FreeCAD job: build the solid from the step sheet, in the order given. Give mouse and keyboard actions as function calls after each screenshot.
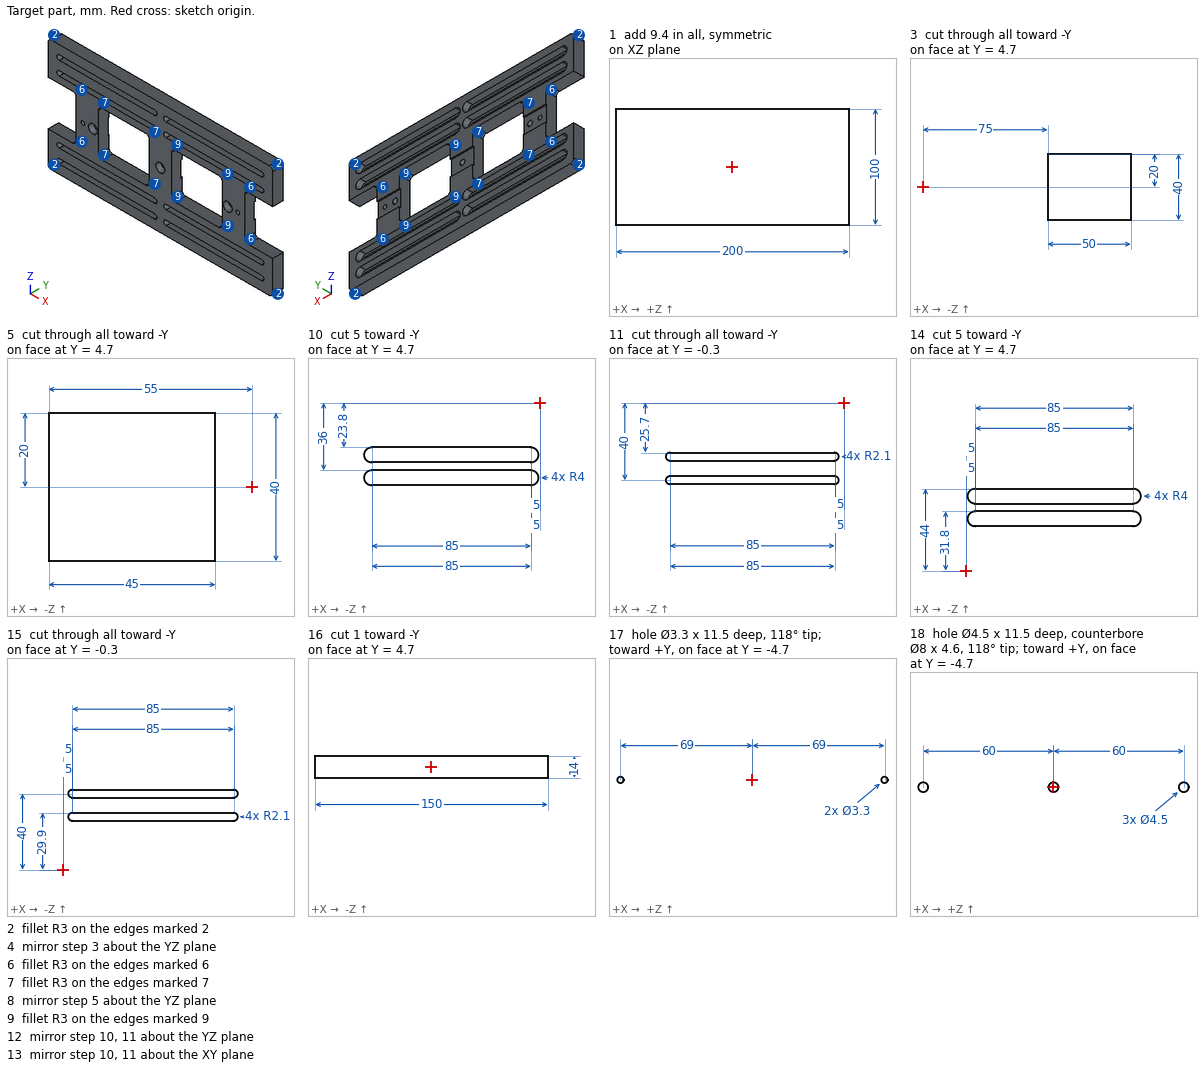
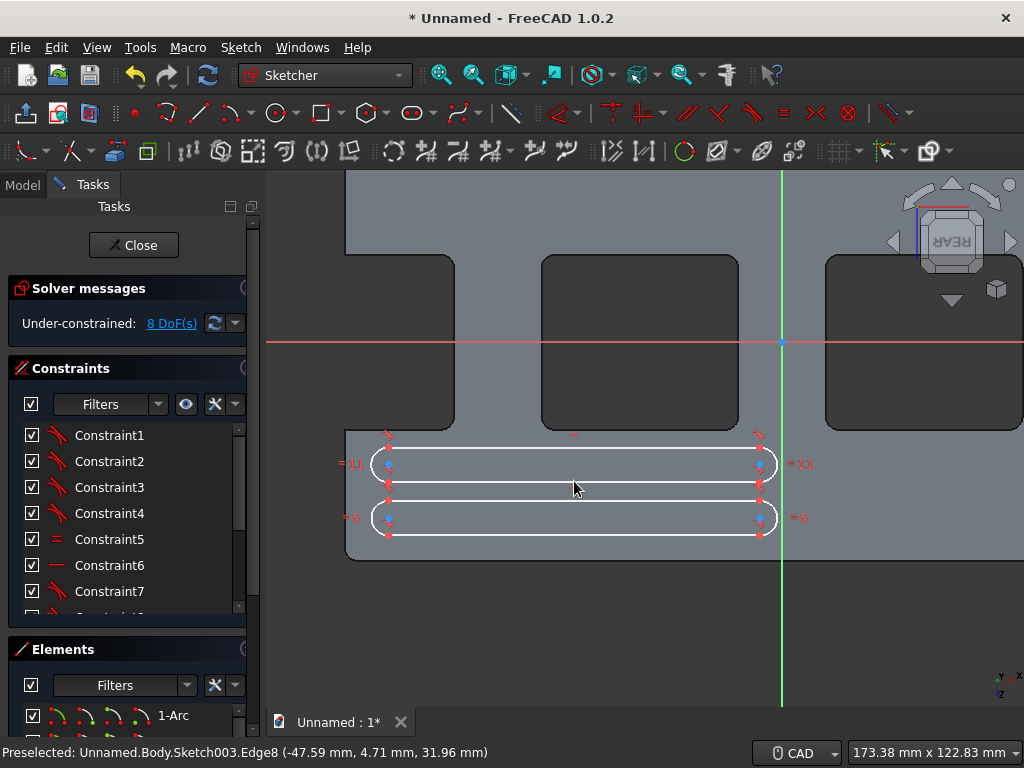
click(375, 508)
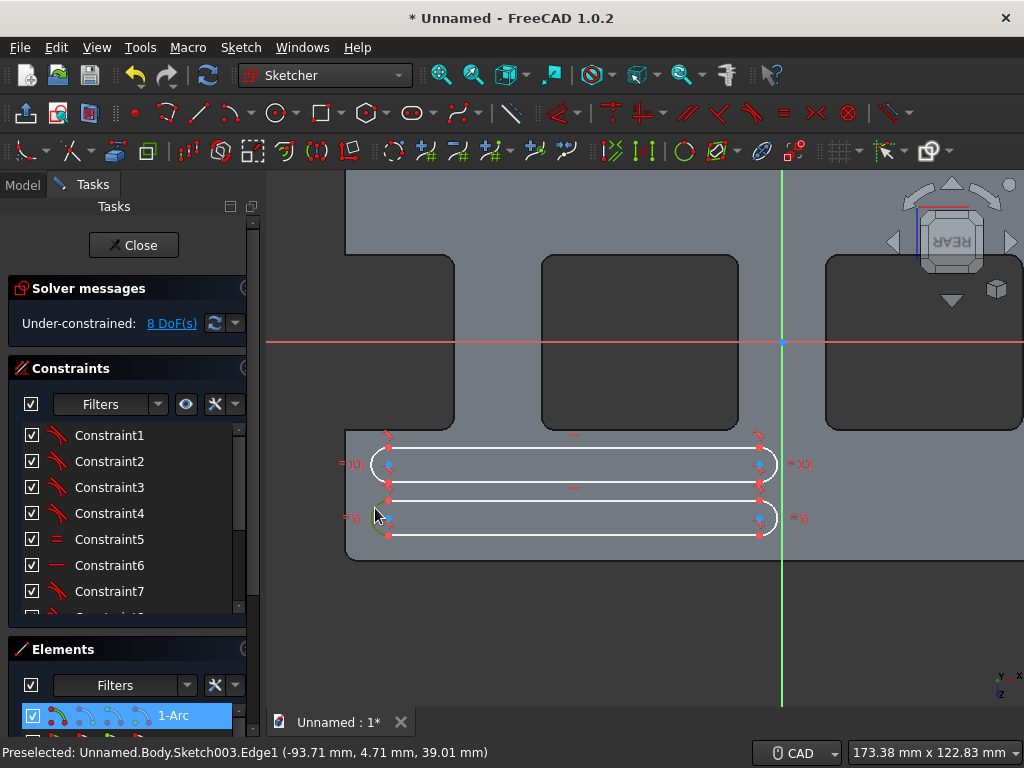
click(375, 455)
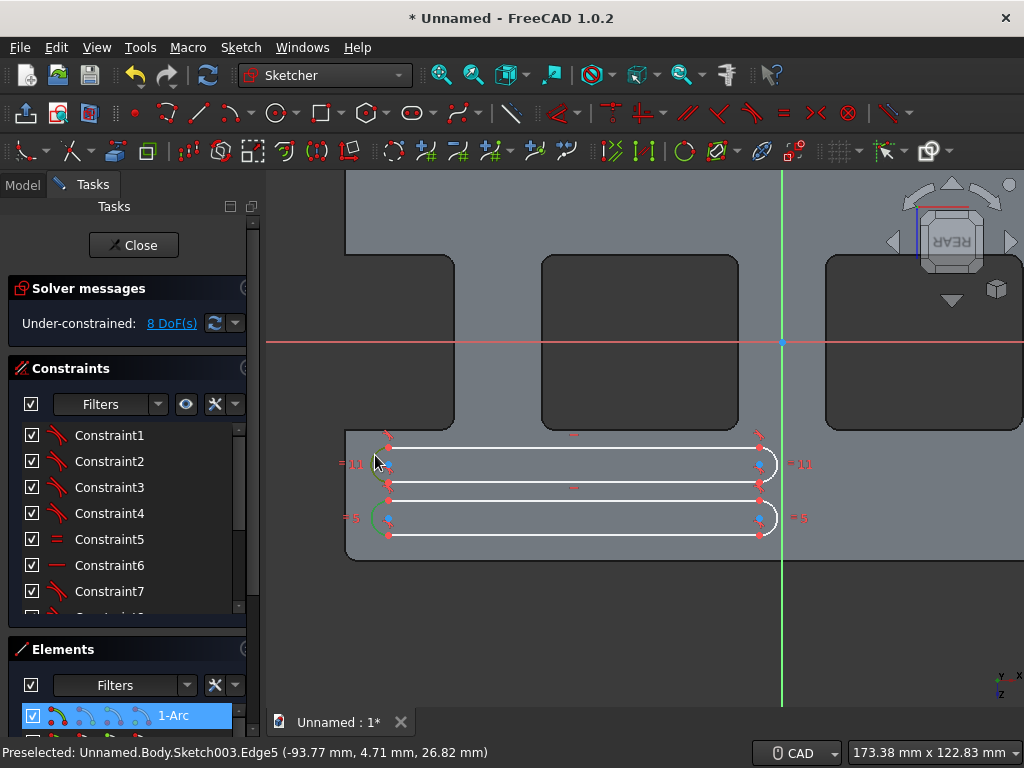
click(784, 114)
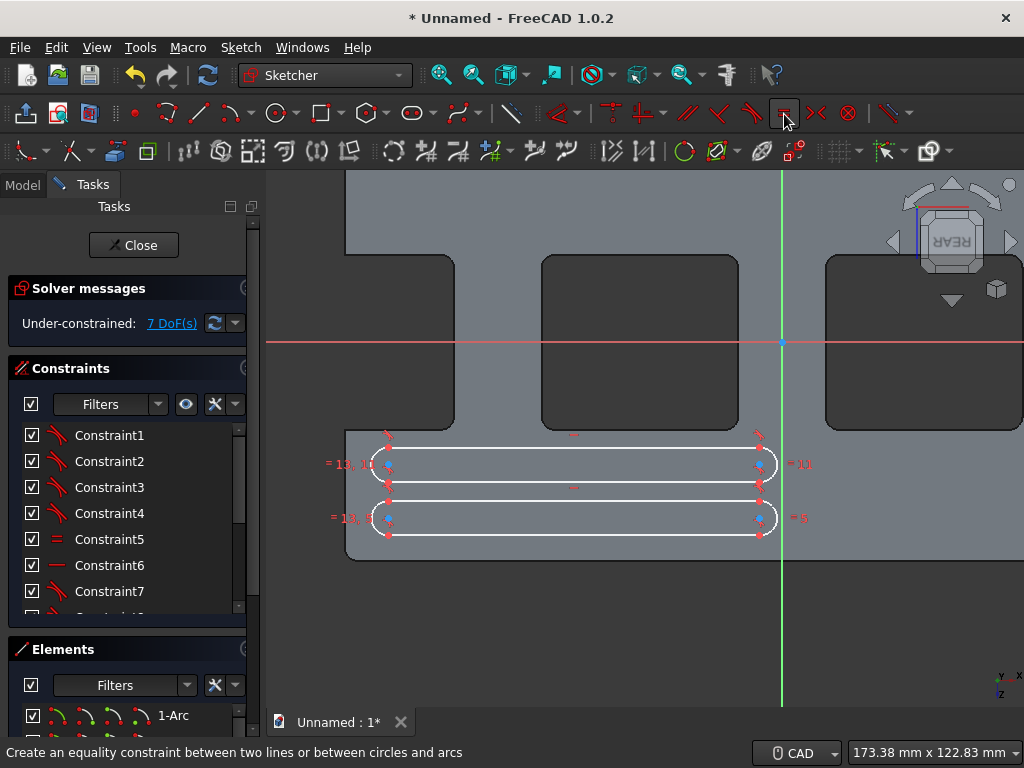
key(d)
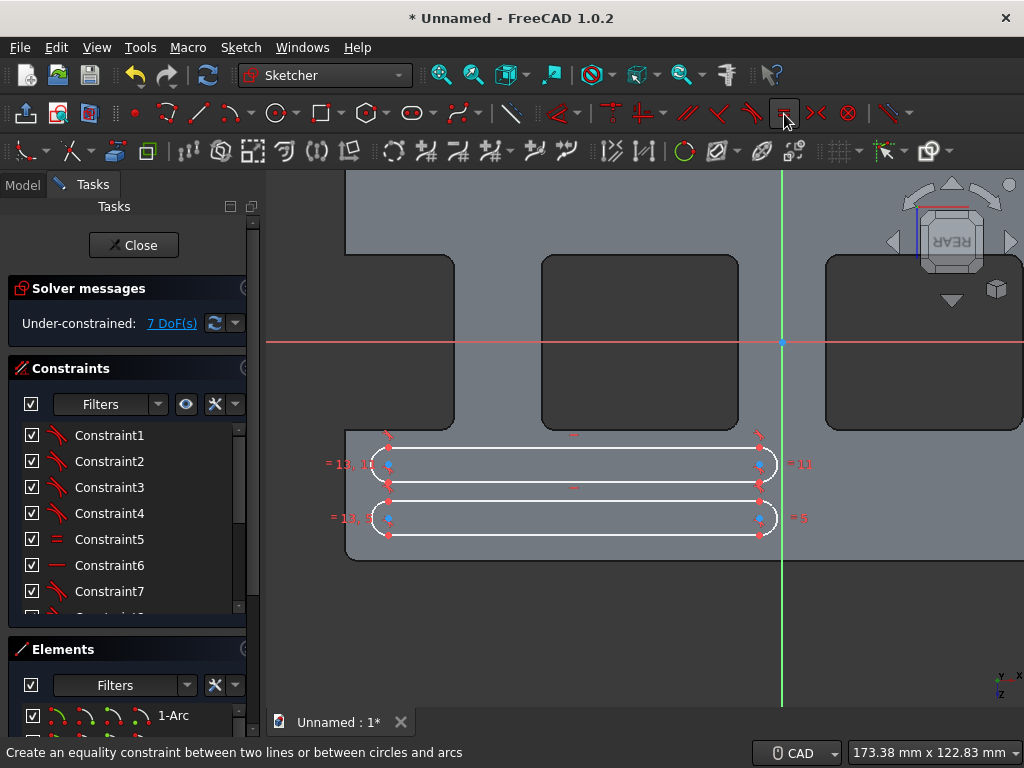
scroll(375, 508, up, 5)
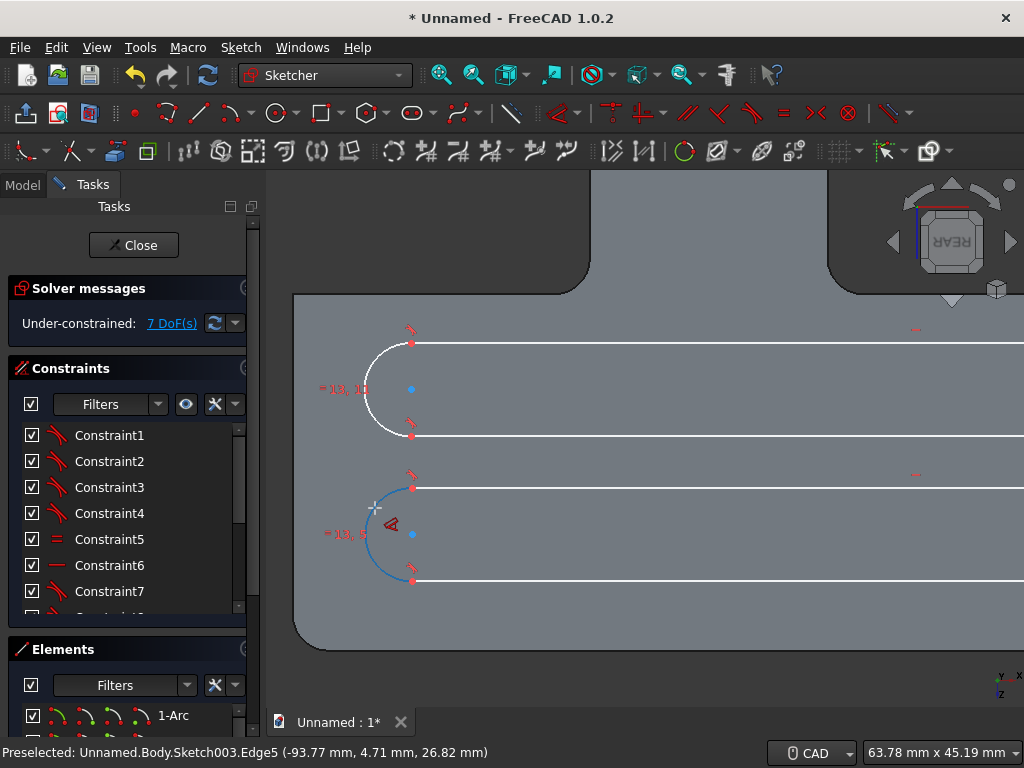
click(374, 507)
click(348, 488)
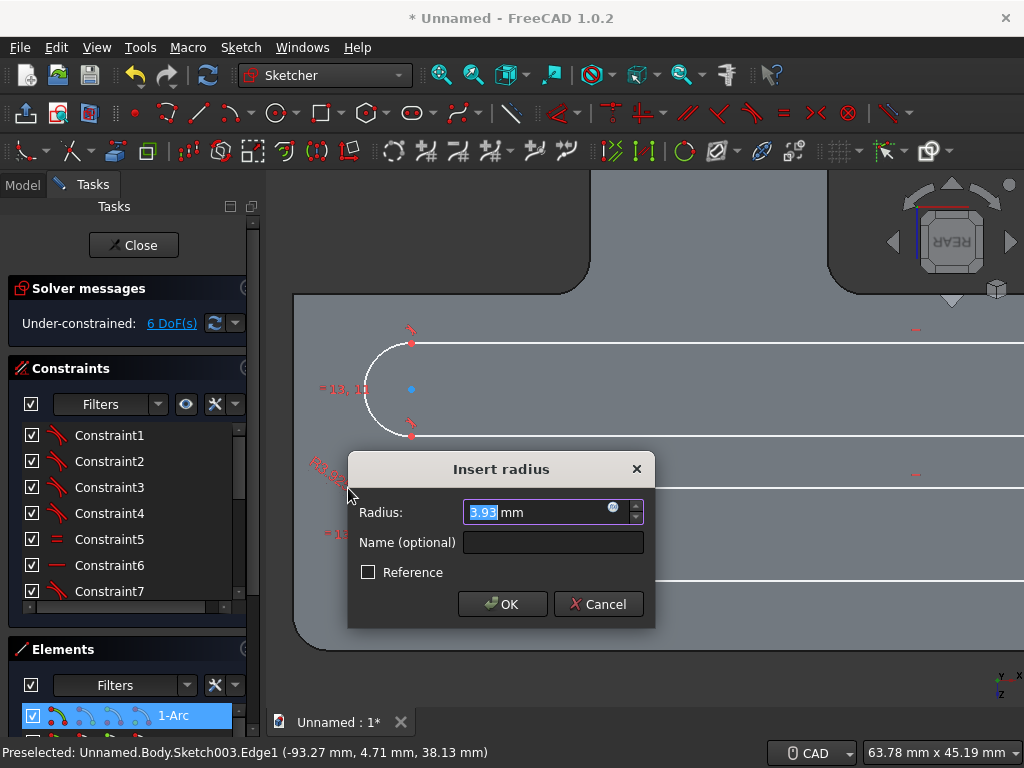
text(4)
key(Return)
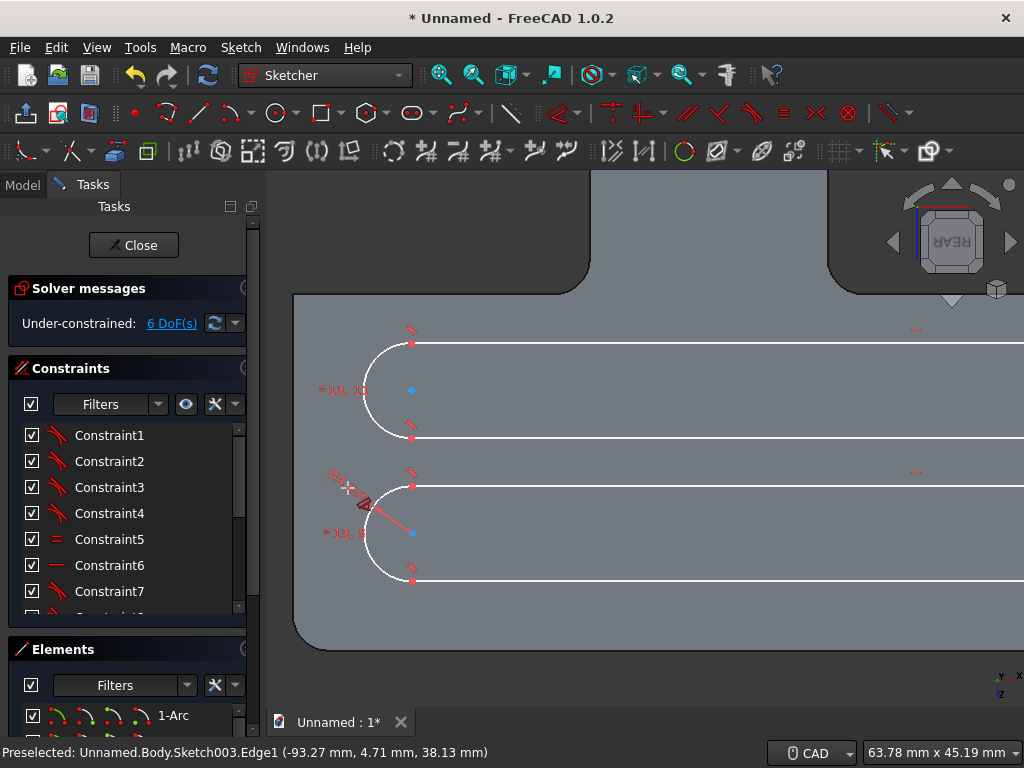
click(715, 486)
click(636, 520)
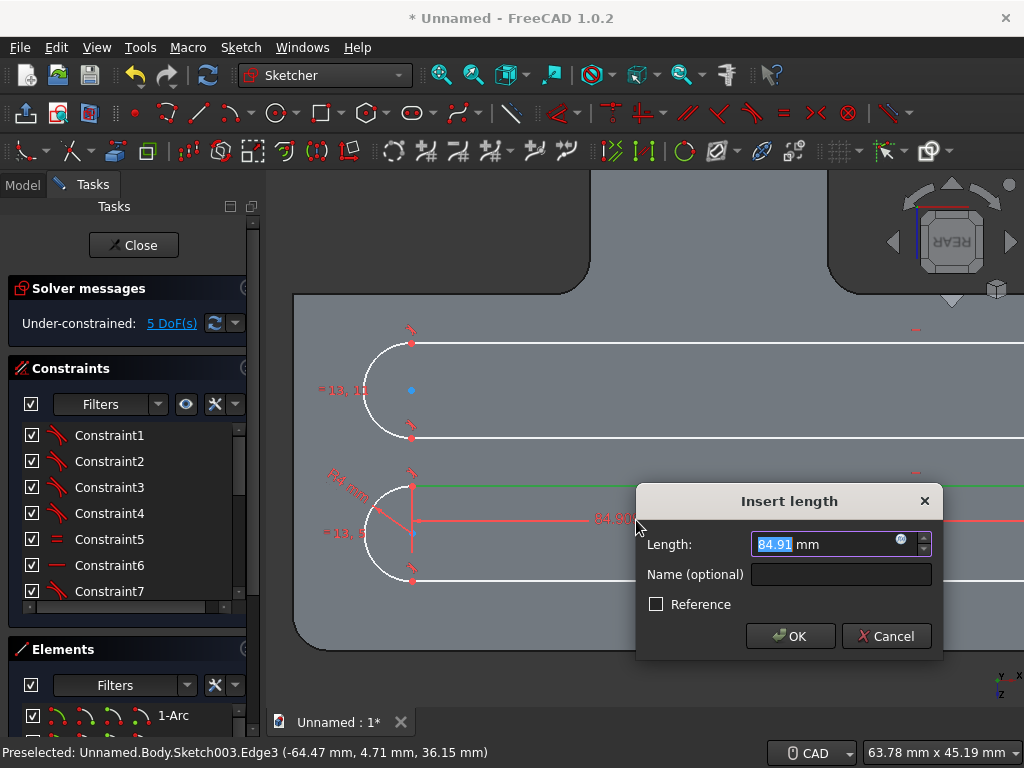
text(85)
key(Return)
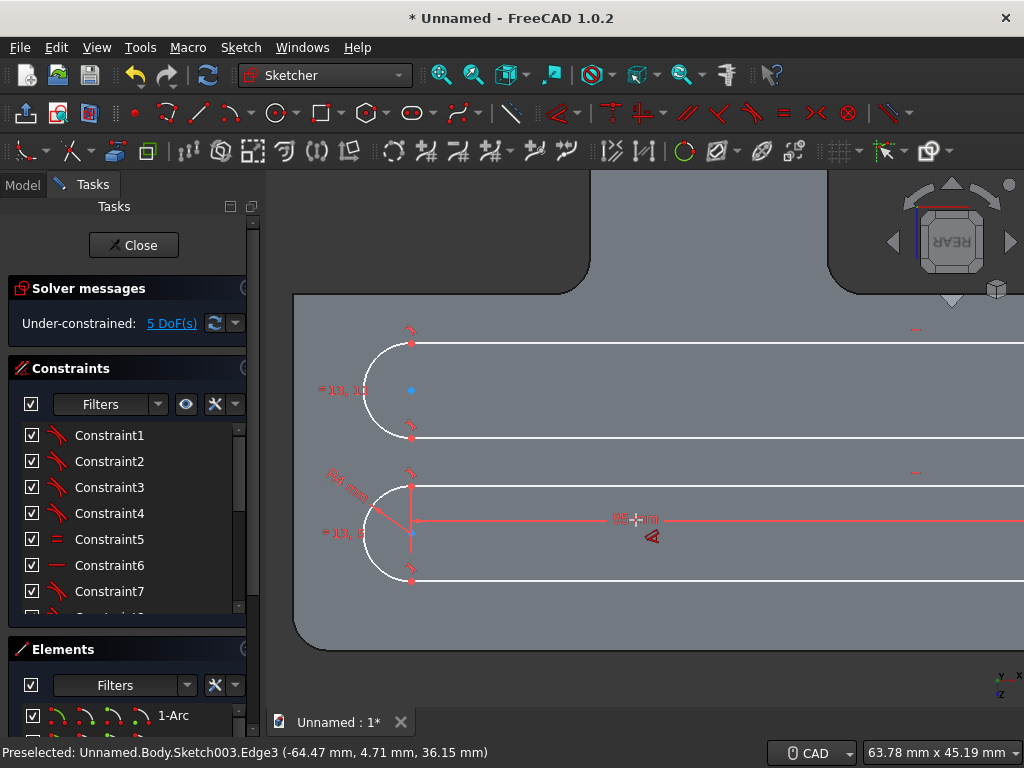
click(714, 343)
click(635, 377)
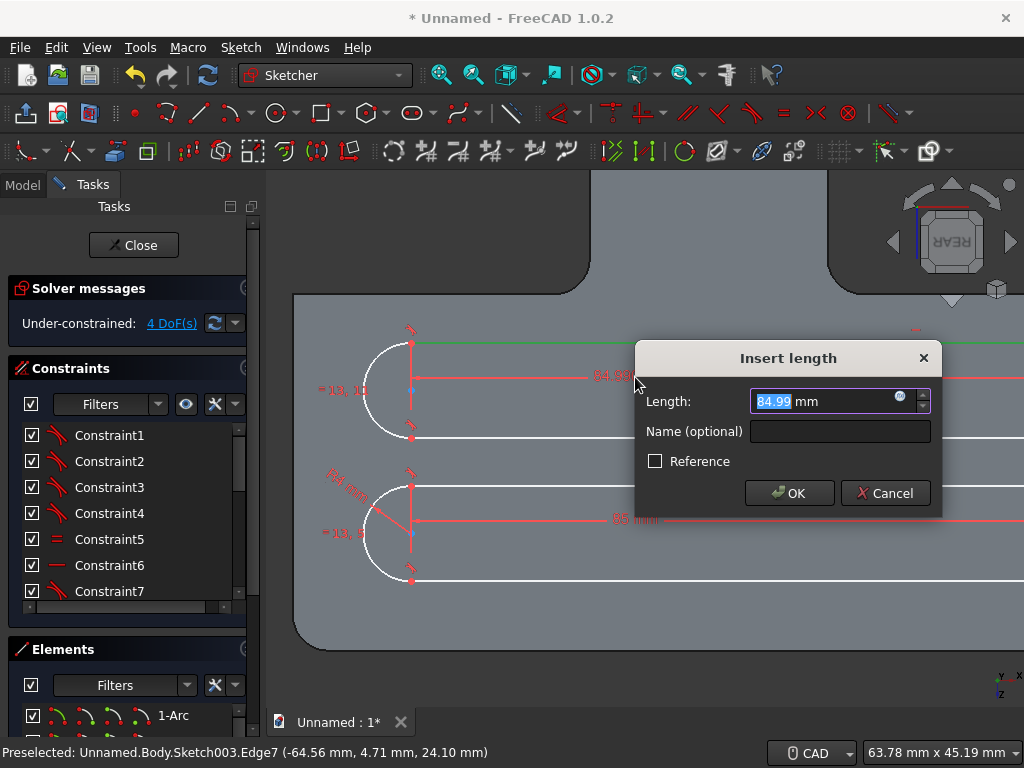
text(85)
key(Return)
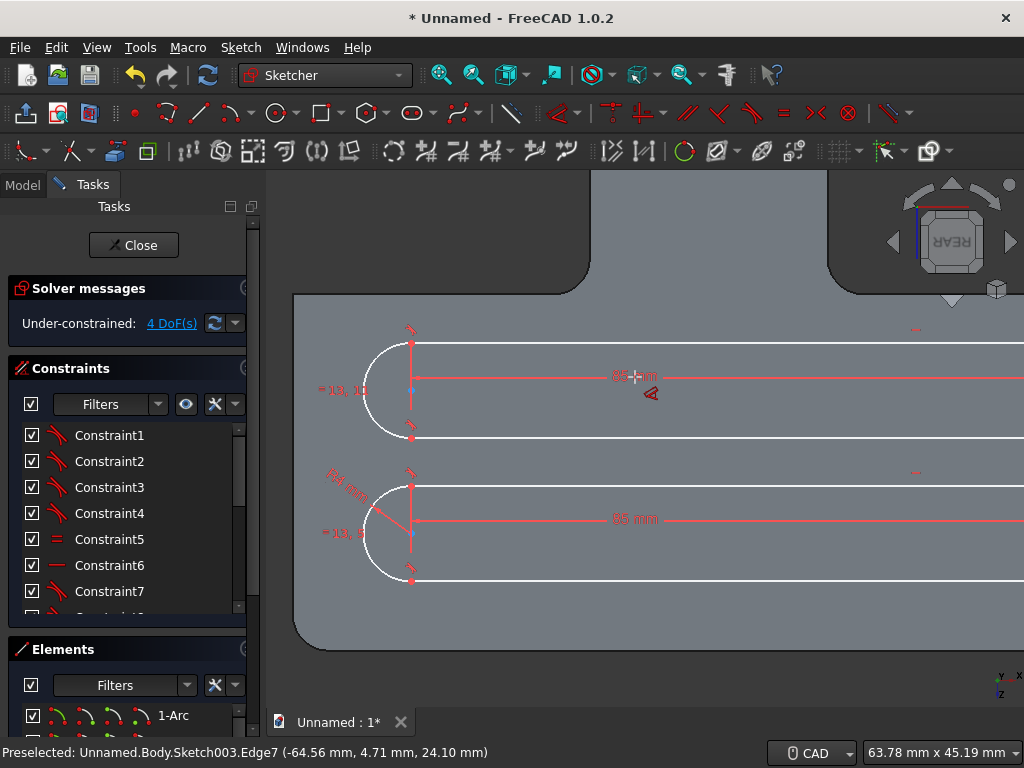
scroll(375, 509, down, 5)